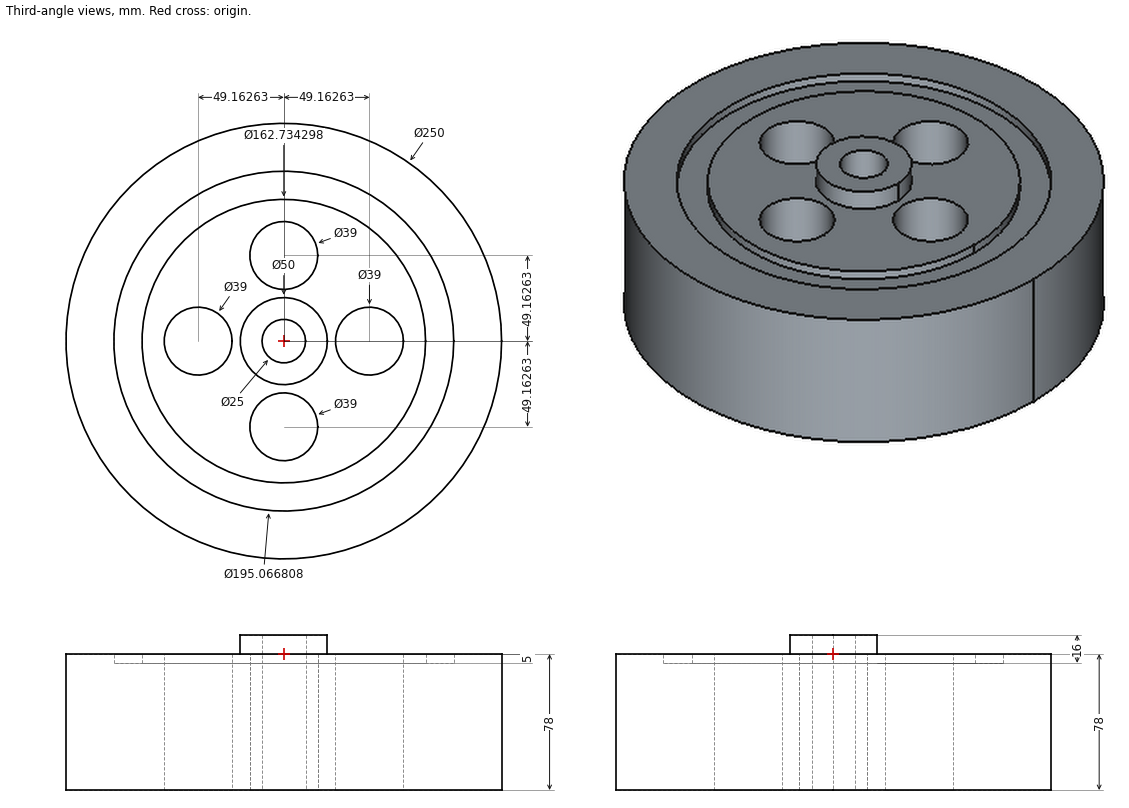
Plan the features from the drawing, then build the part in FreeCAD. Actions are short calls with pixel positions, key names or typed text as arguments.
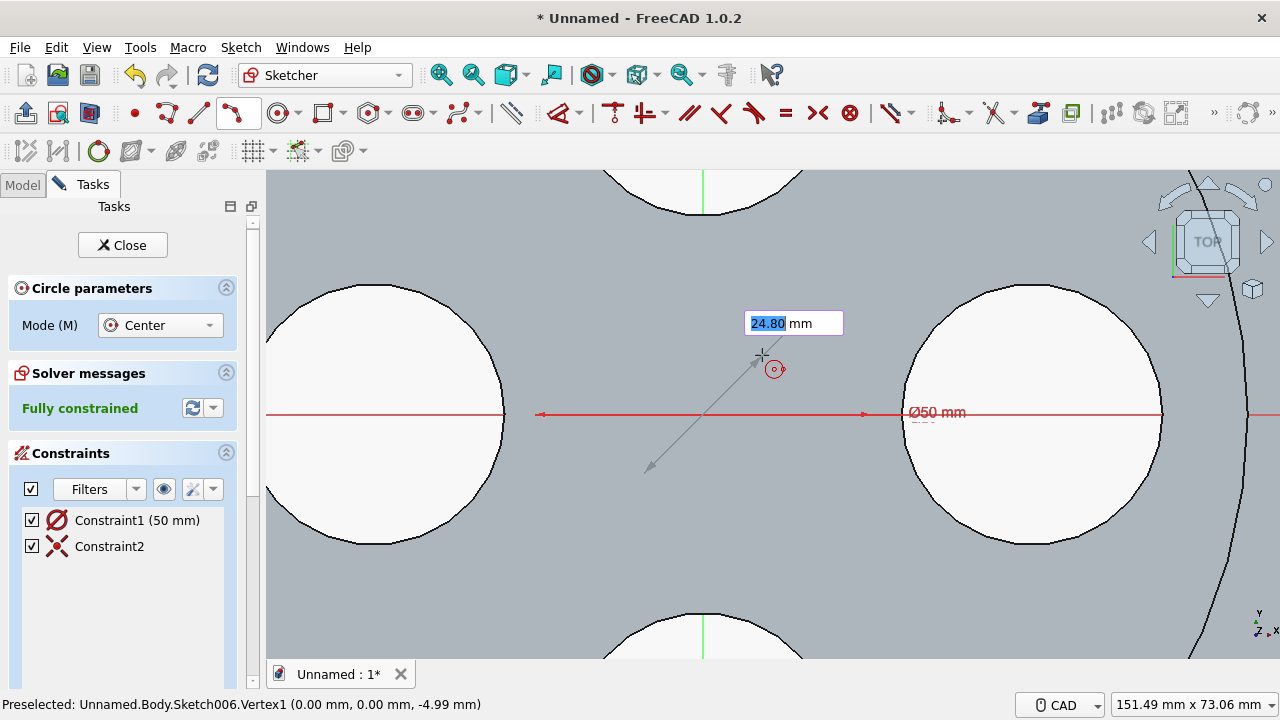
text(25)
key(Return)
key(Escape)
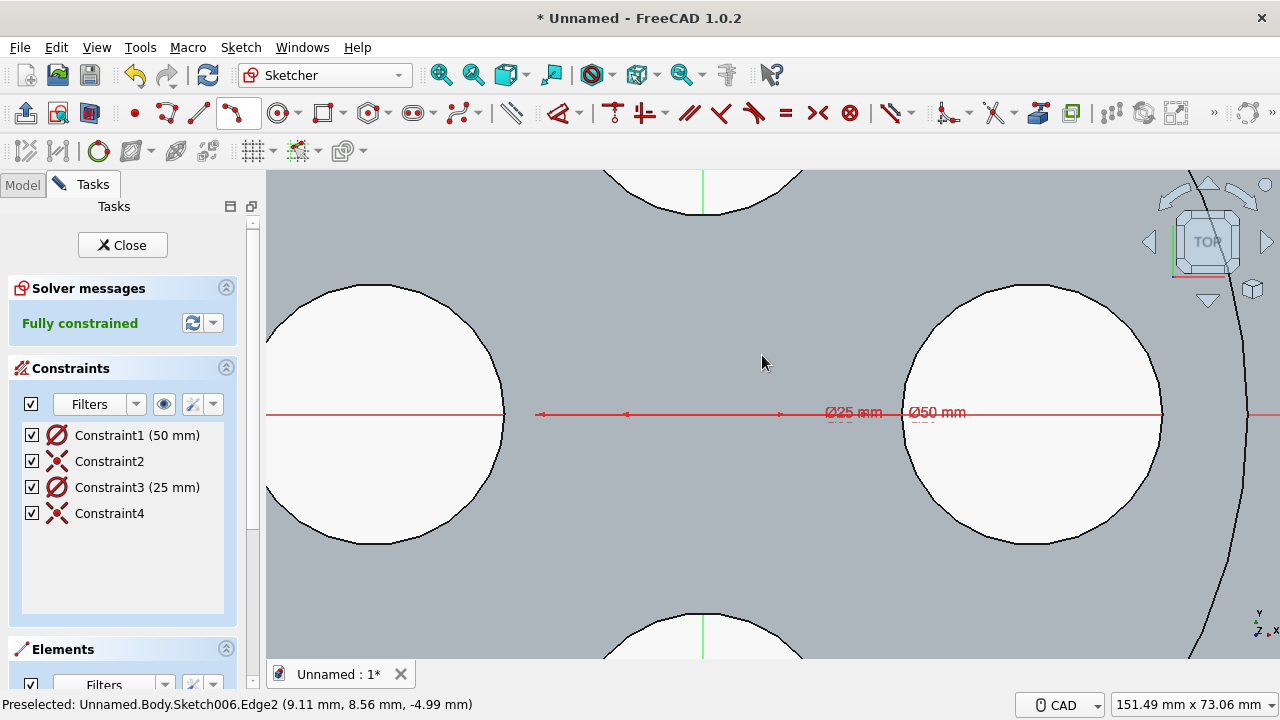
click(123, 245)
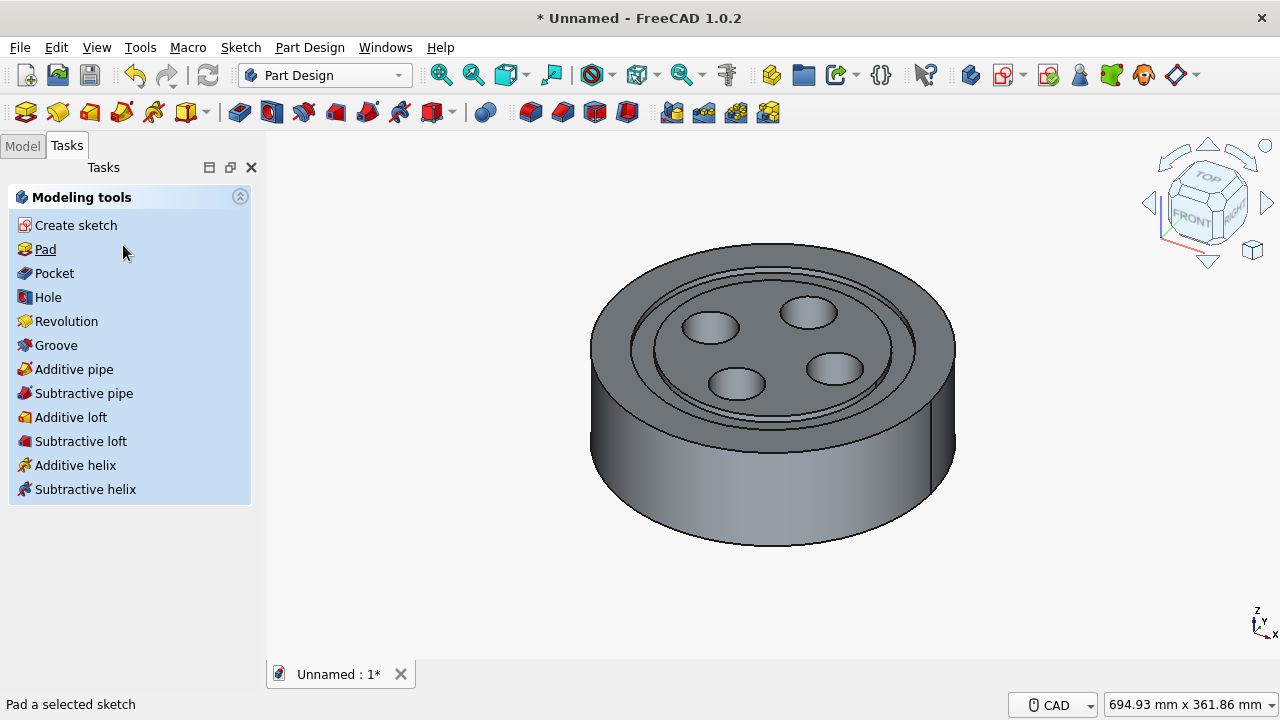
click(26, 112)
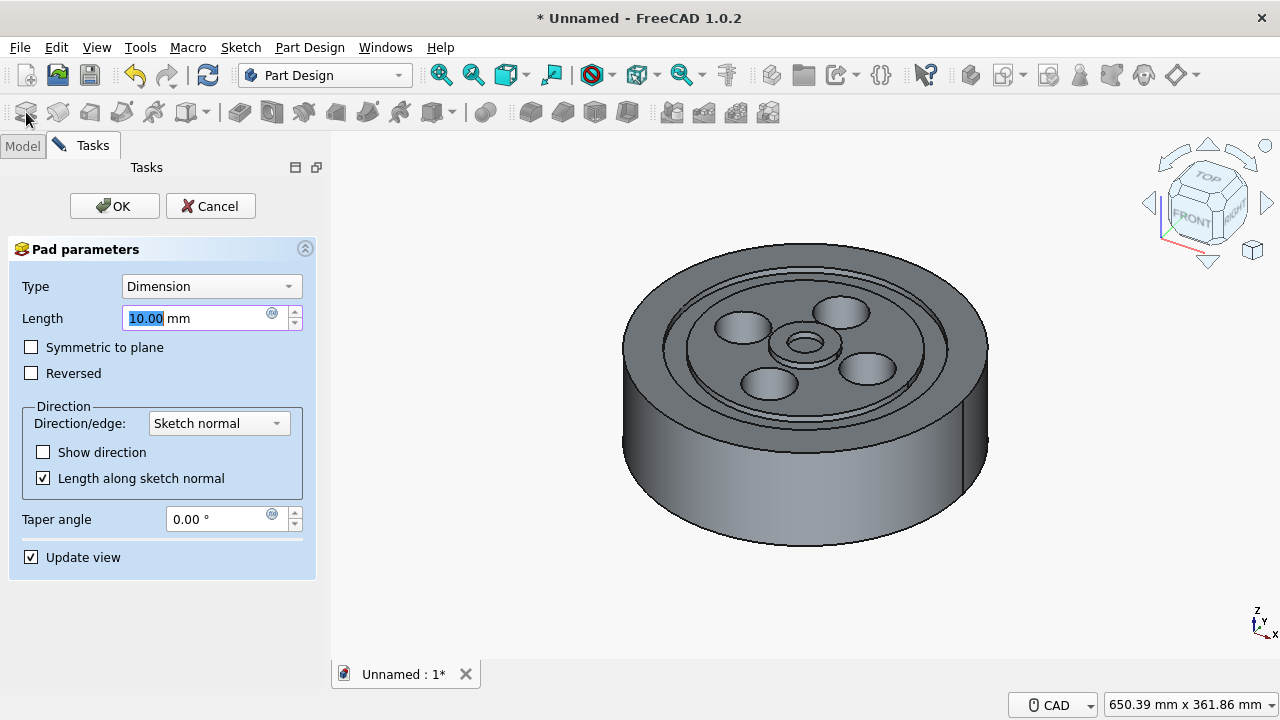
text(16)
key(Tab)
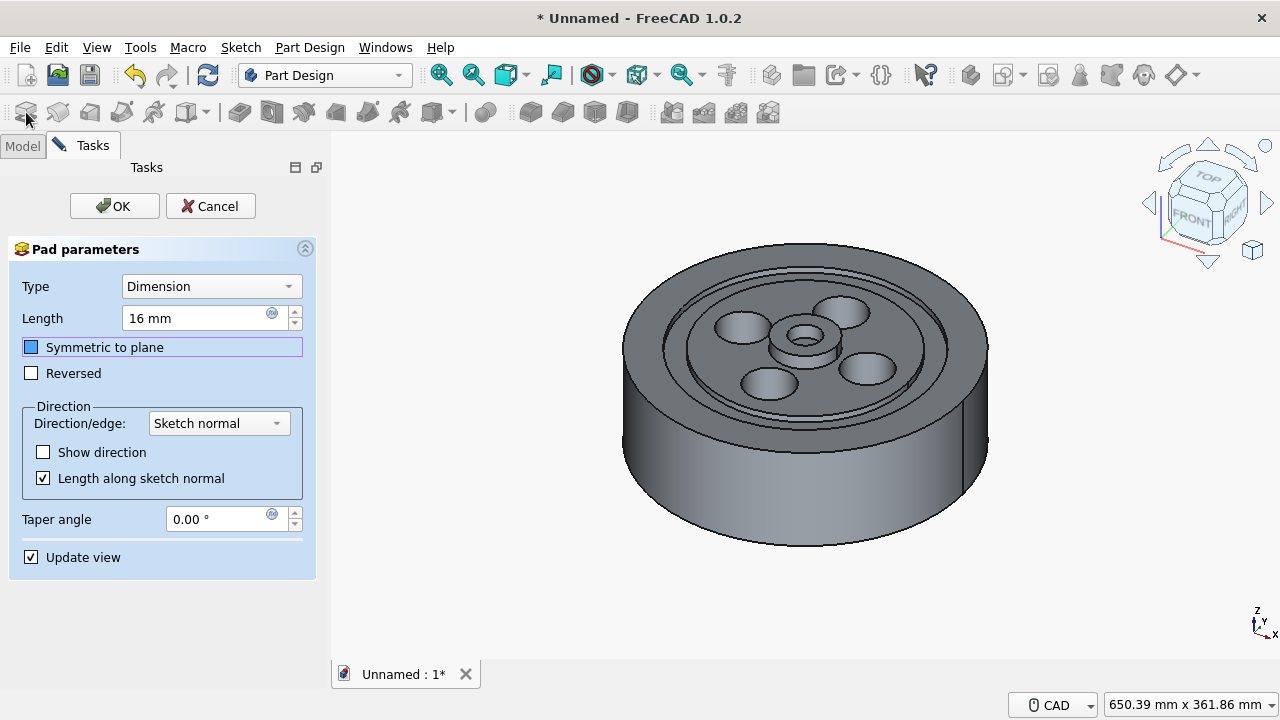
click(115, 206)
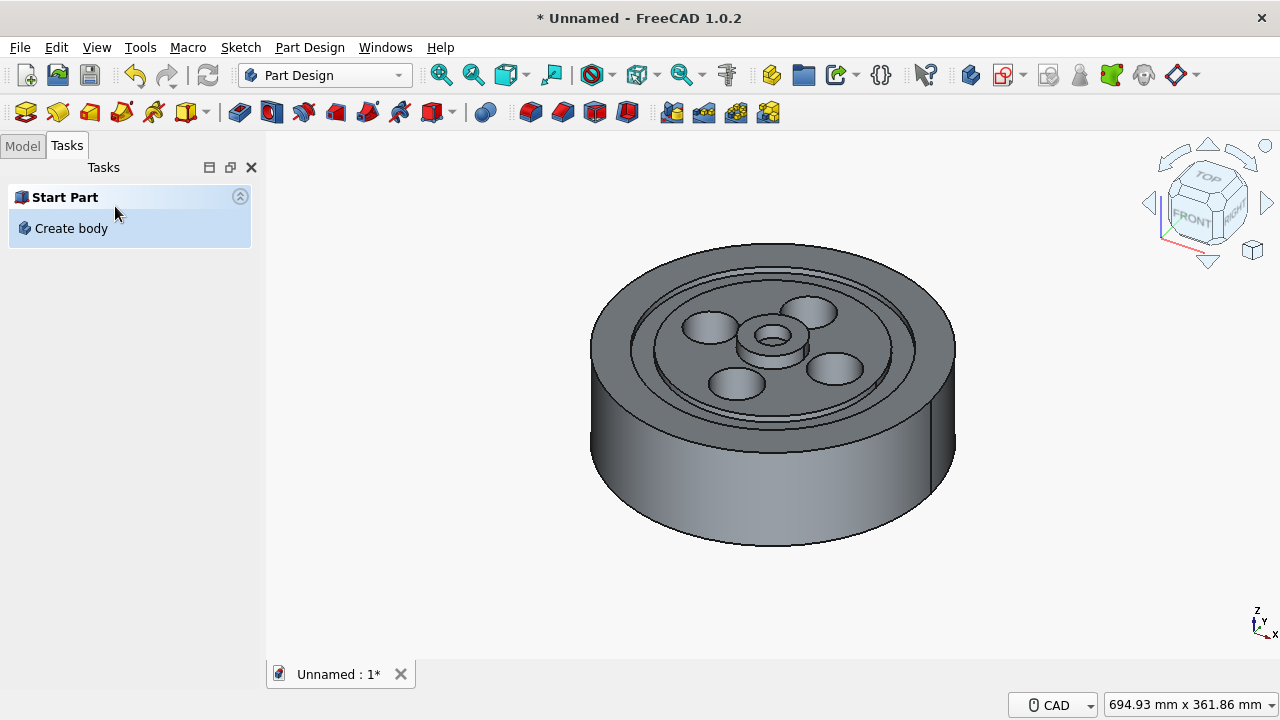
key(5)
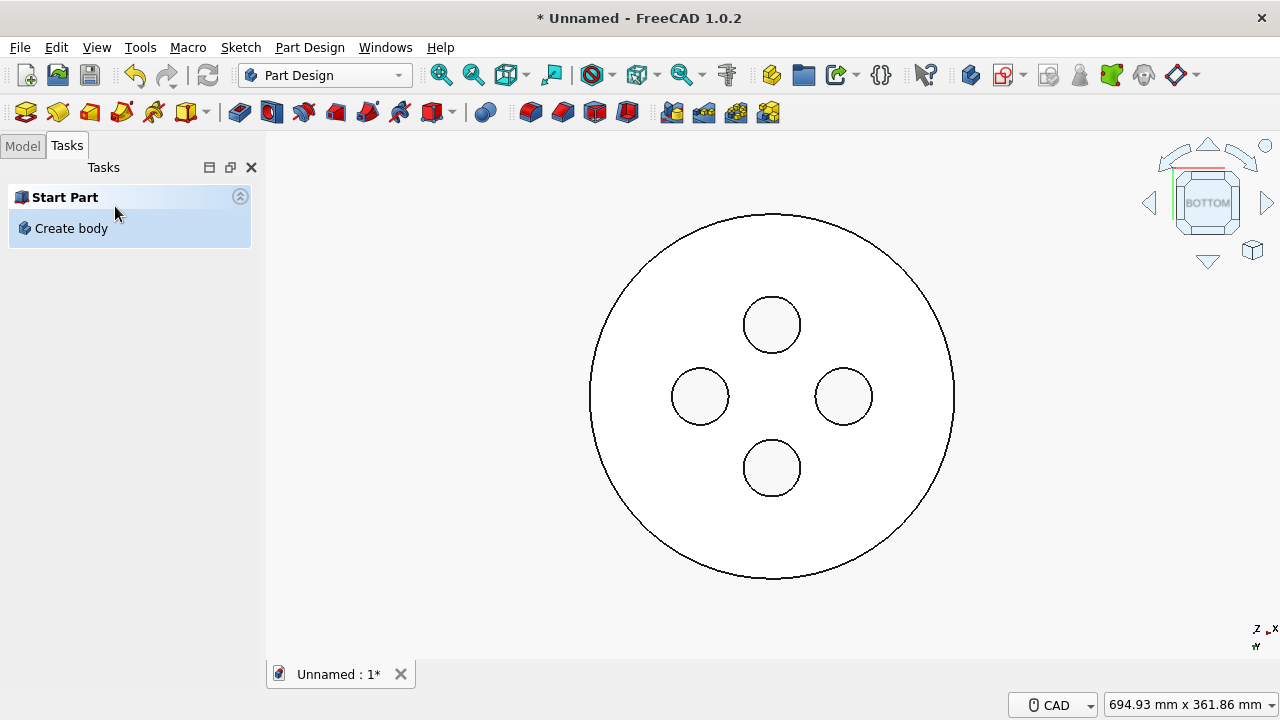
click(772, 395)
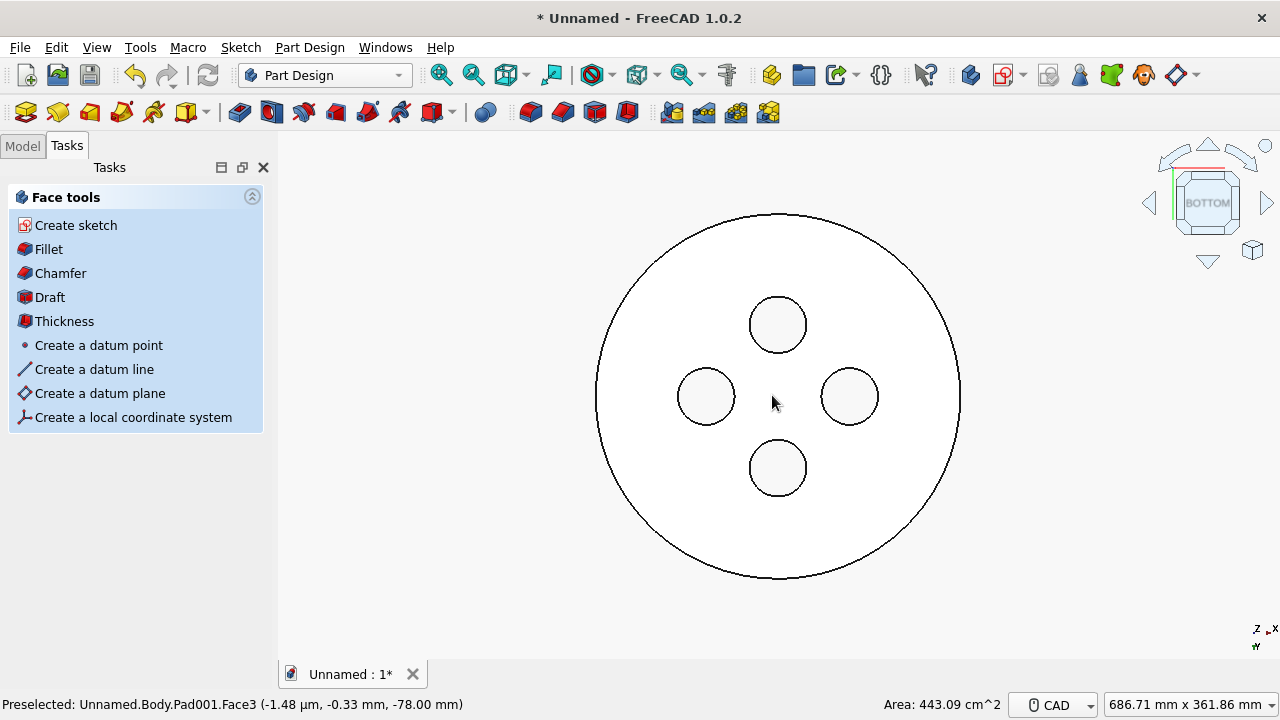
click(1004, 76)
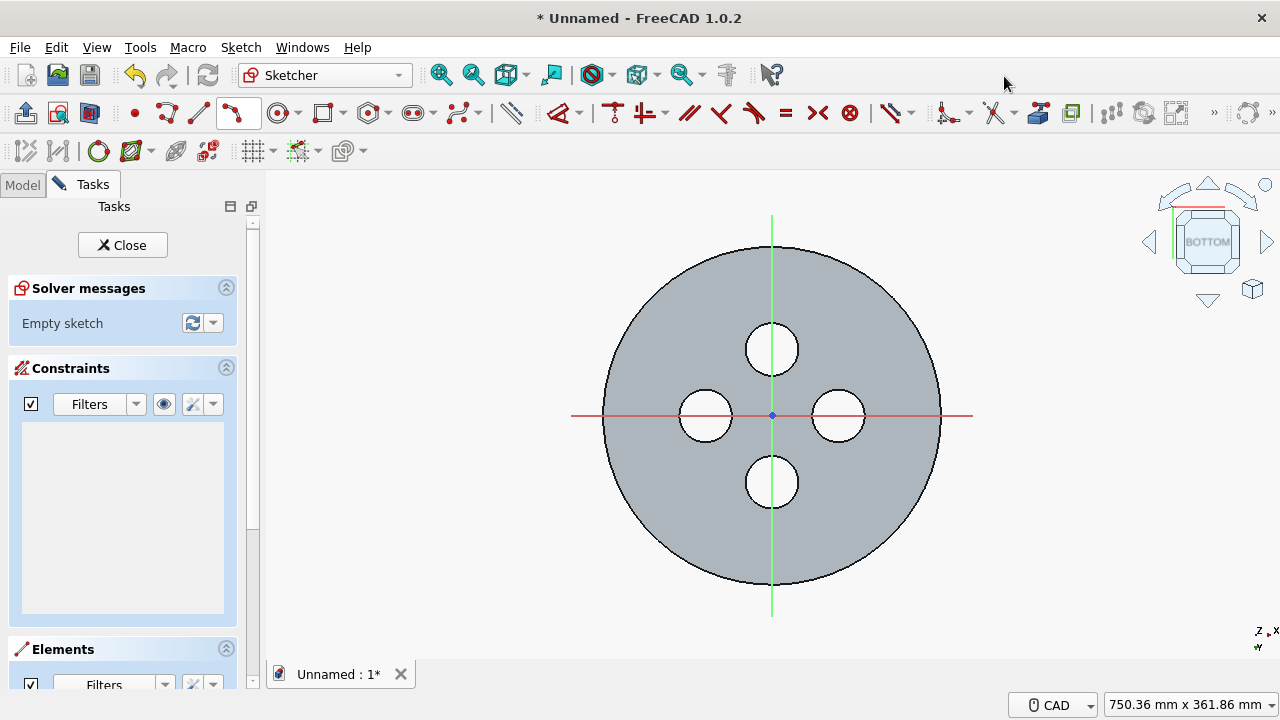
scroll(780, 416, up, 11)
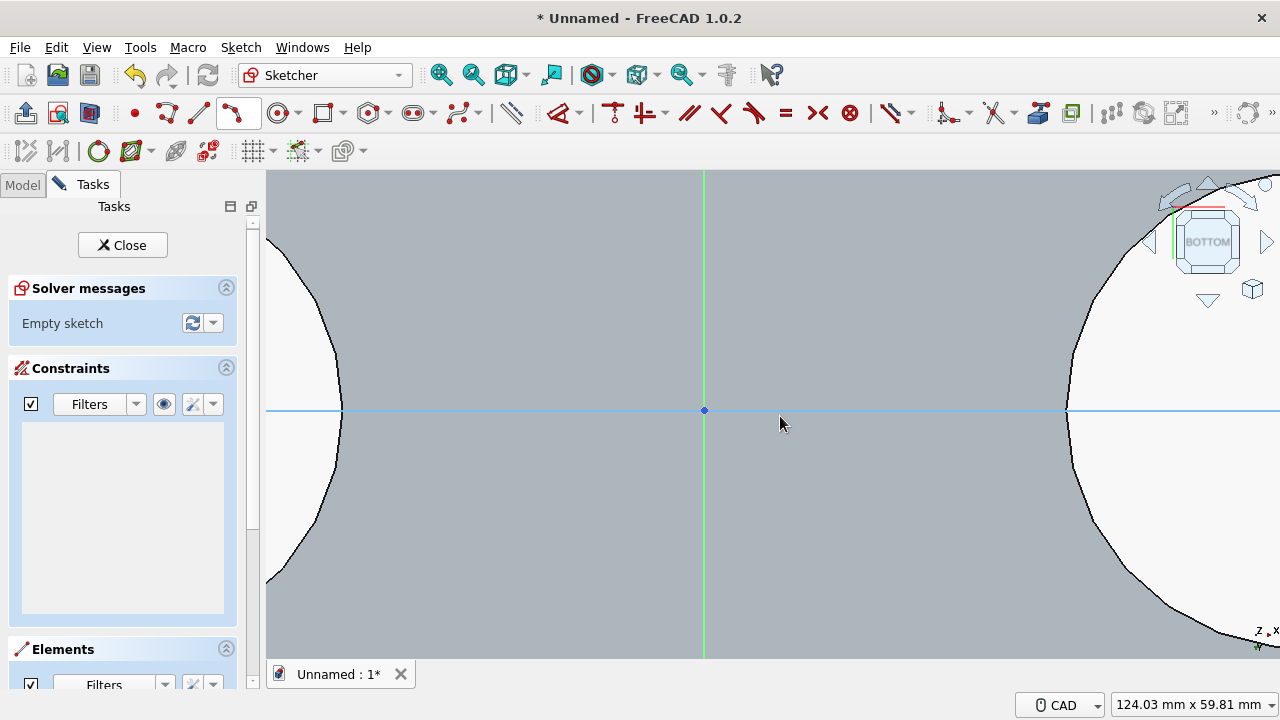
key(g)
key(c)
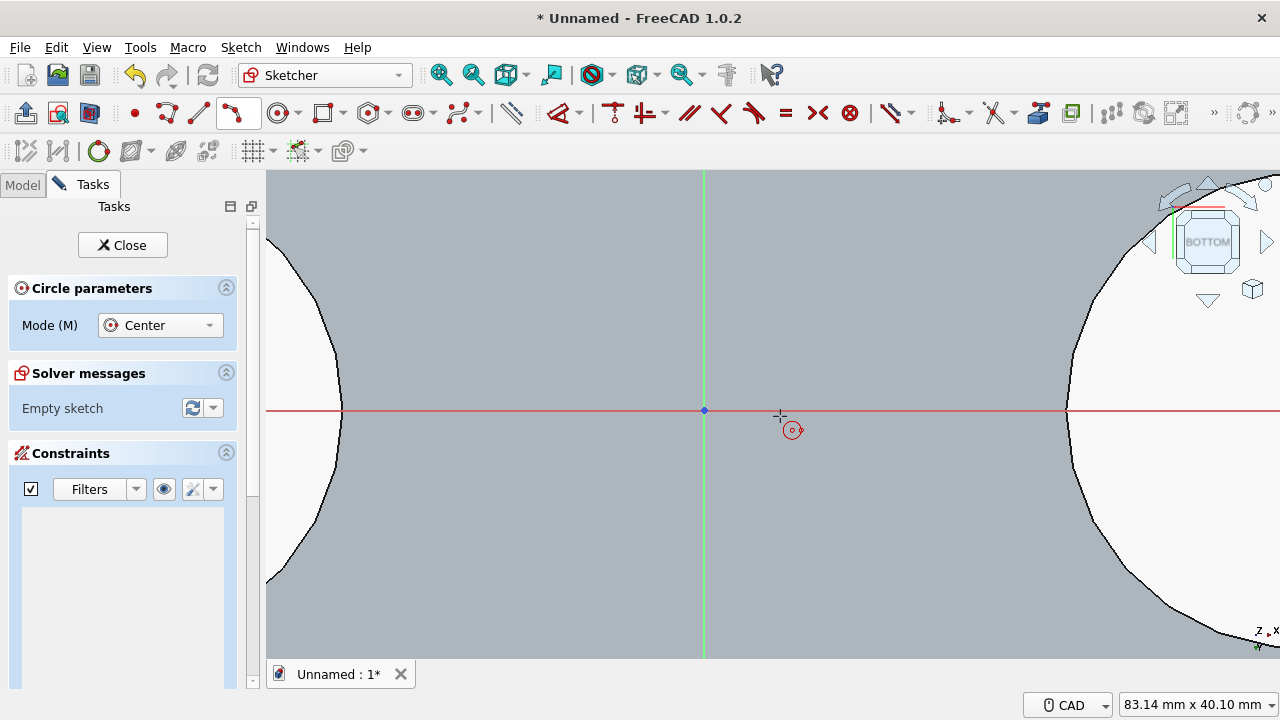
click(704, 411)
move(812, 303)